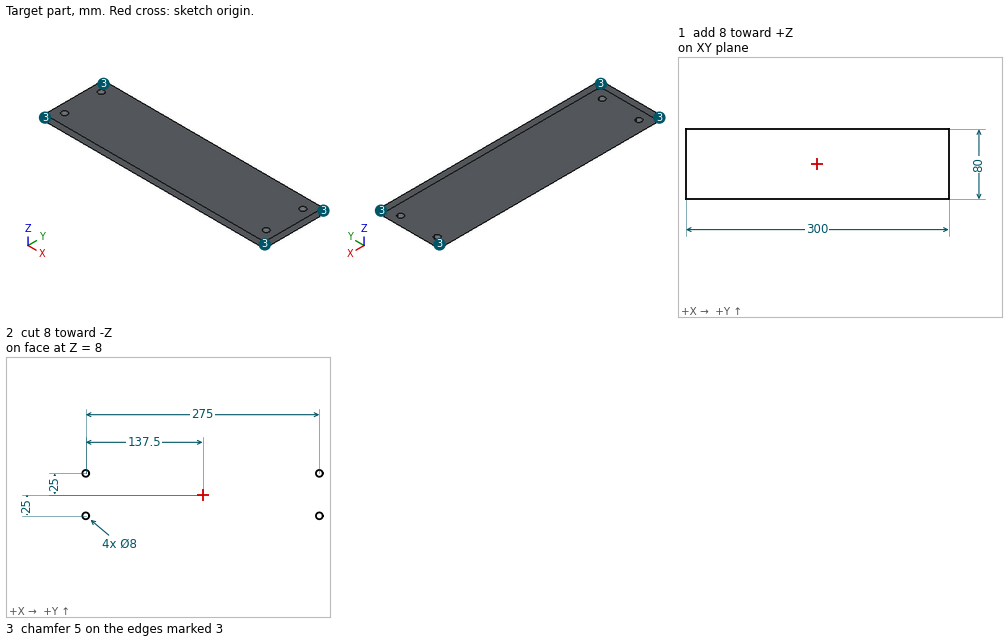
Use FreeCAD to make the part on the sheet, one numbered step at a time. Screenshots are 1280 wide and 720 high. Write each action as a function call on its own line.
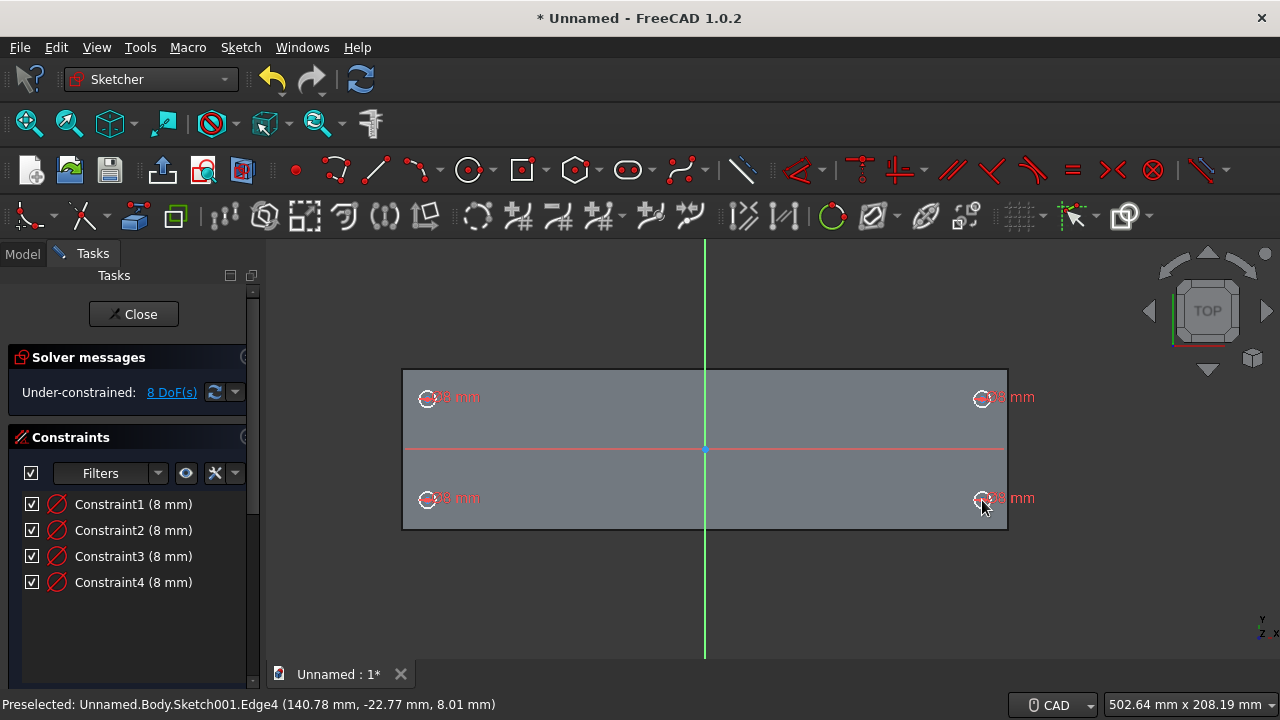
click(428, 399)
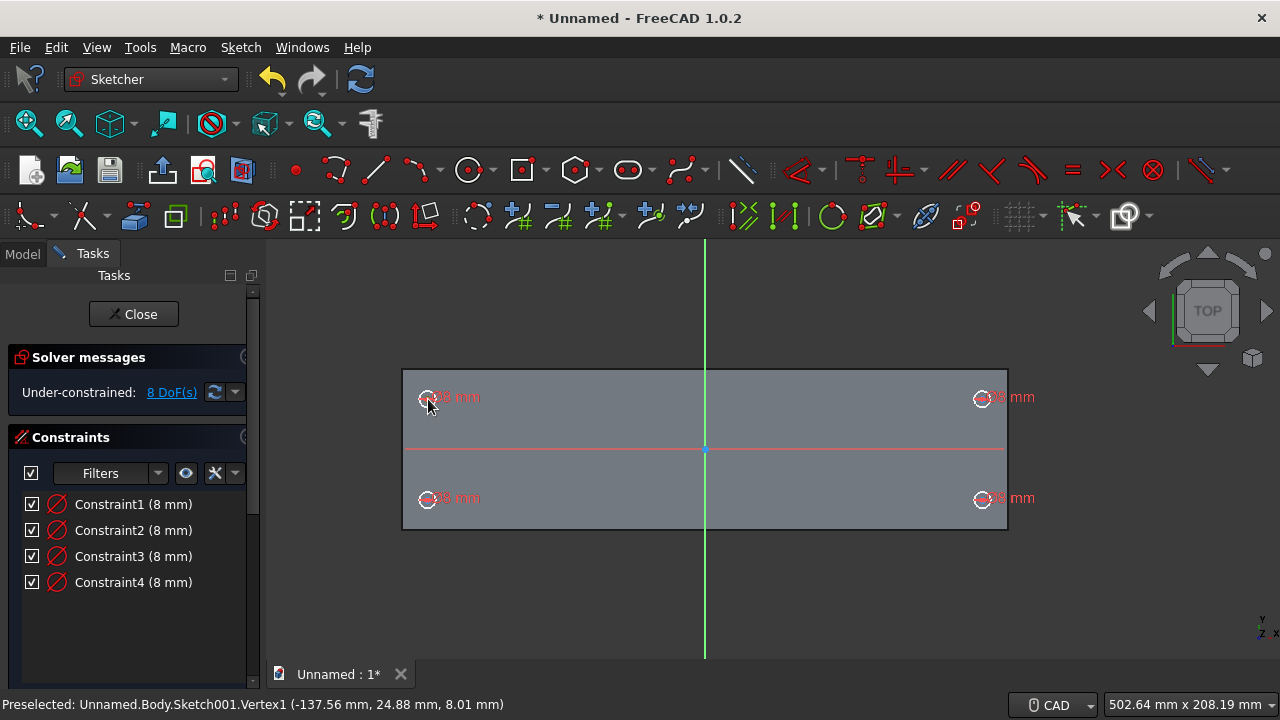
click(428, 500)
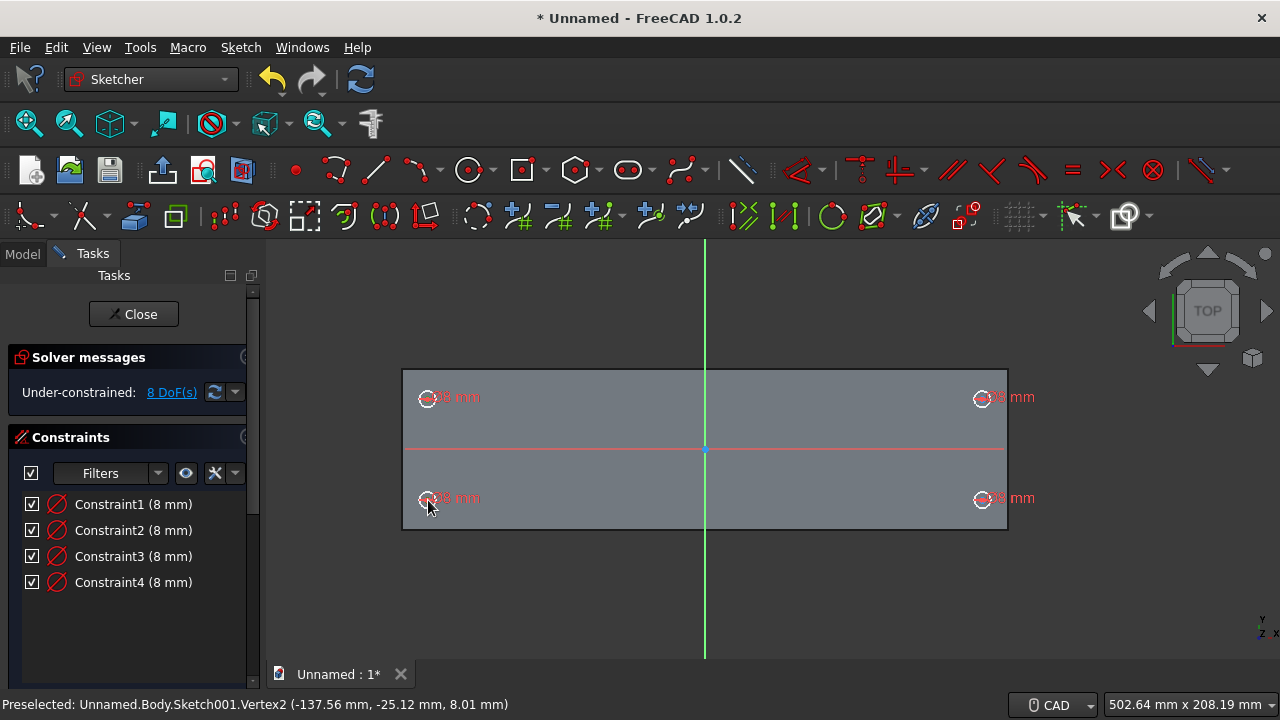
key(v)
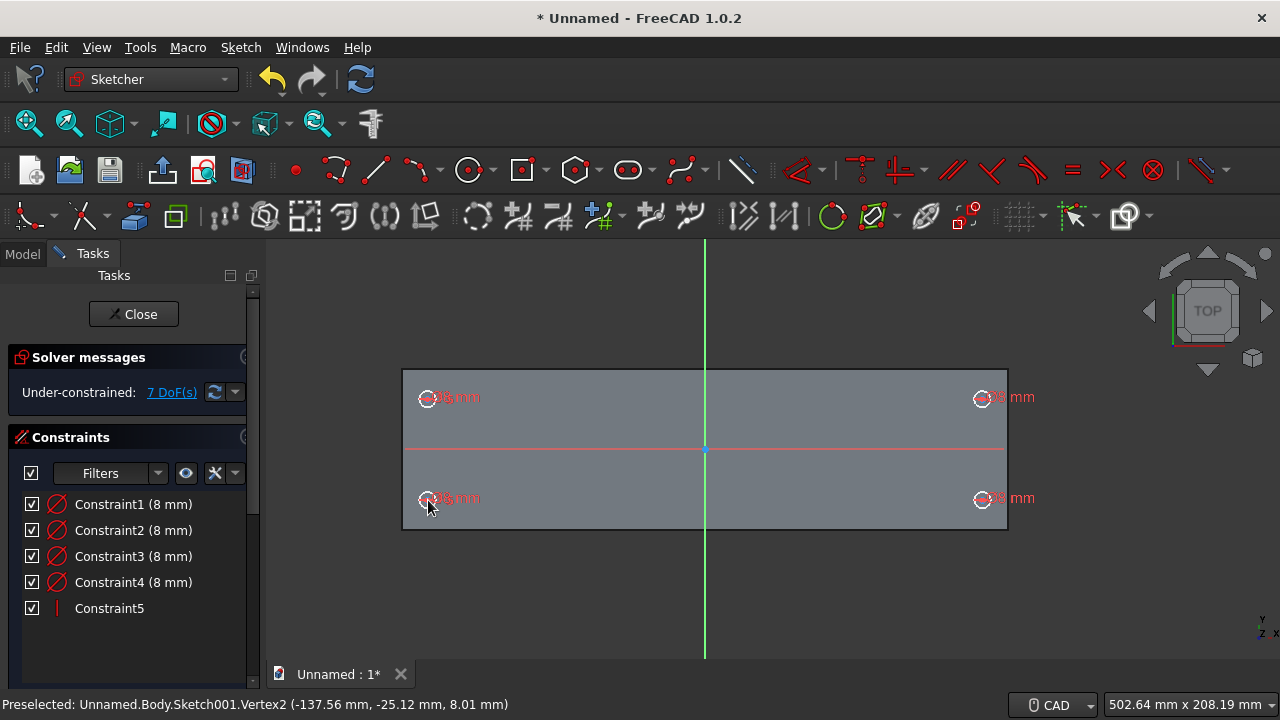
click(428, 399)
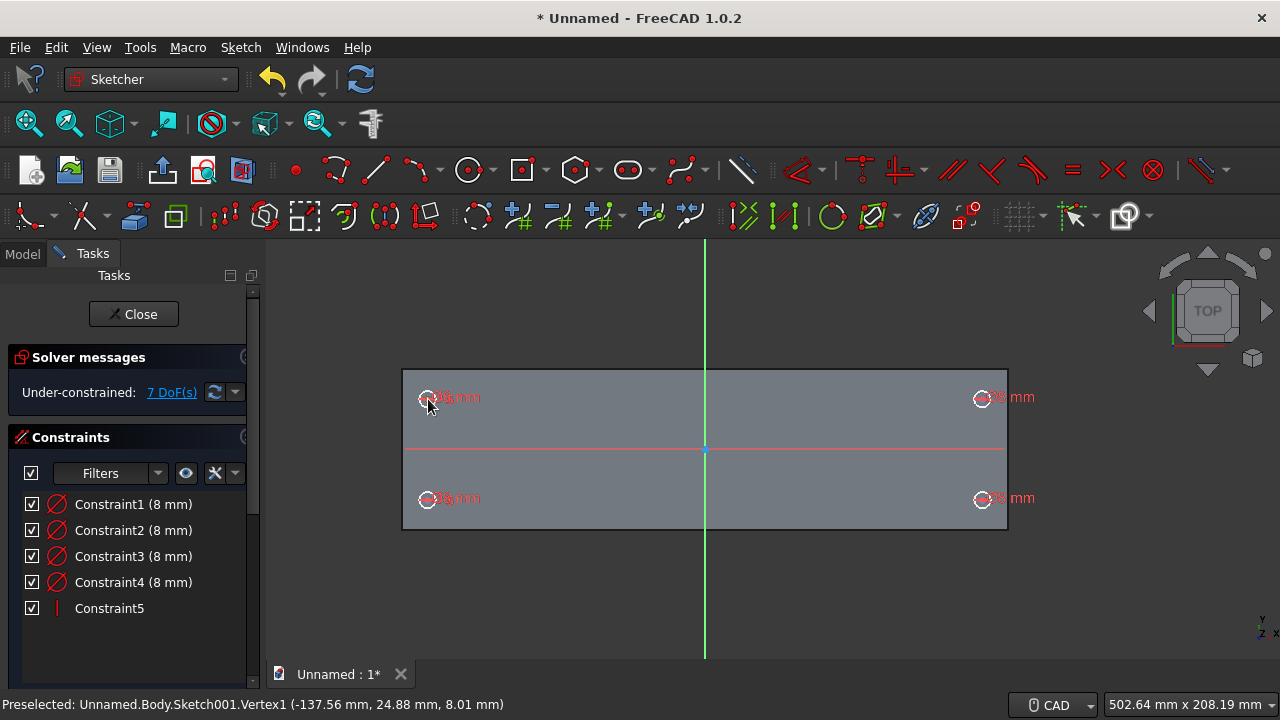
click(982, 399)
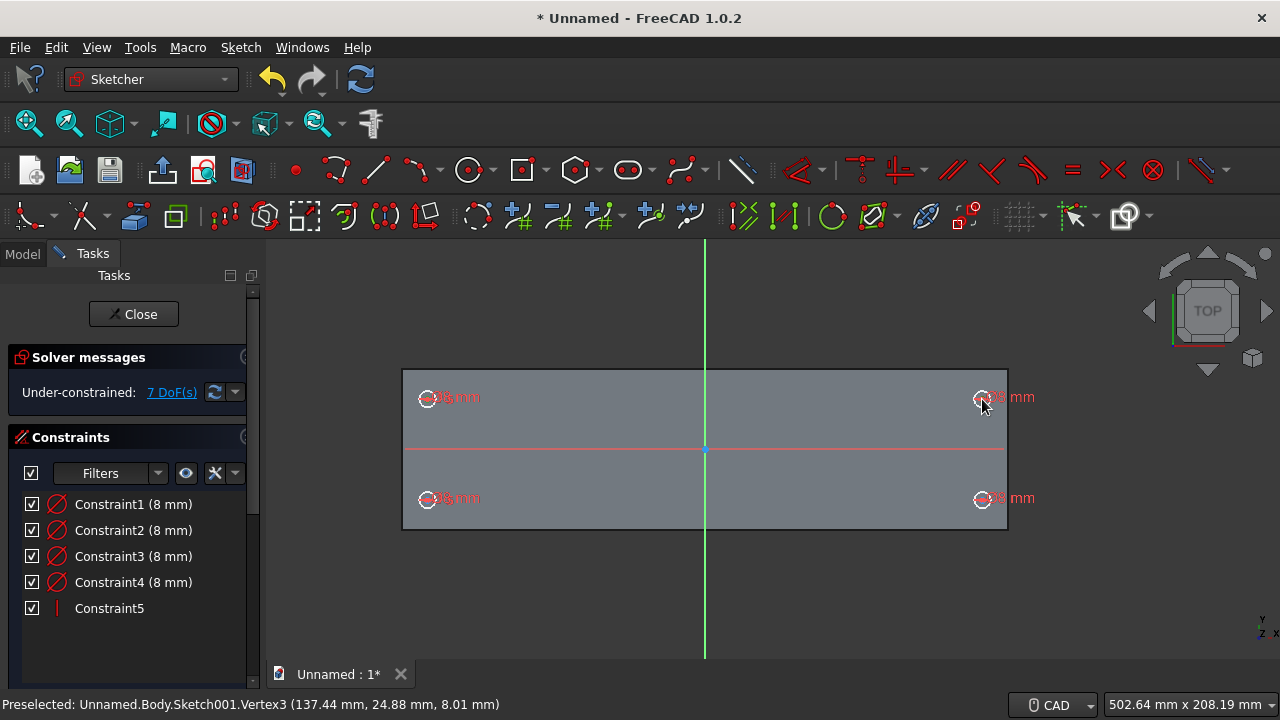
key(h)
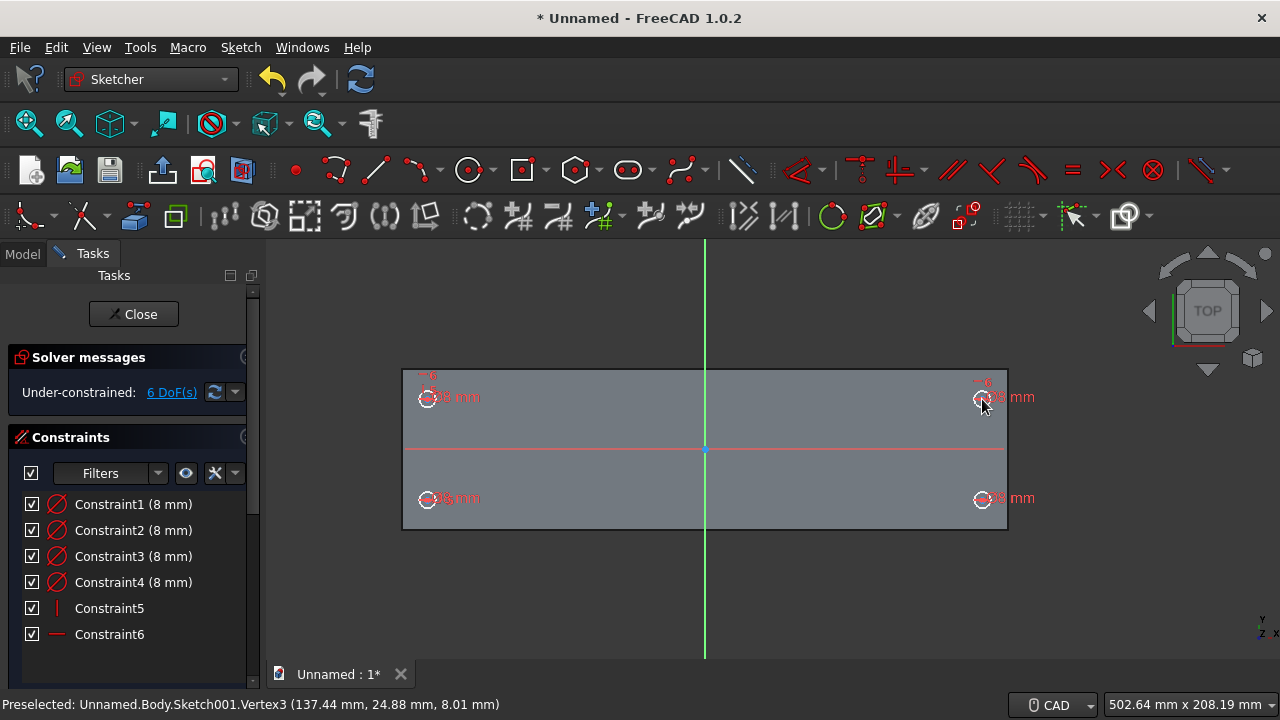
click(982, 399)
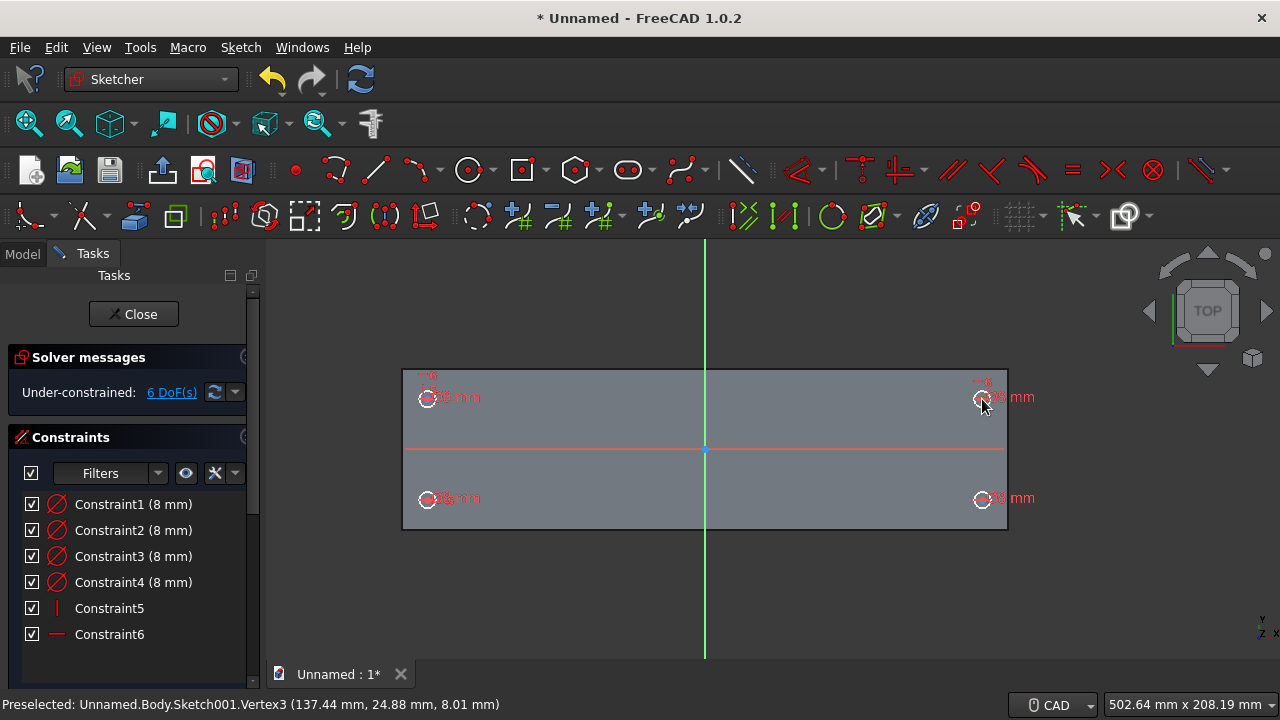
click(982, 500)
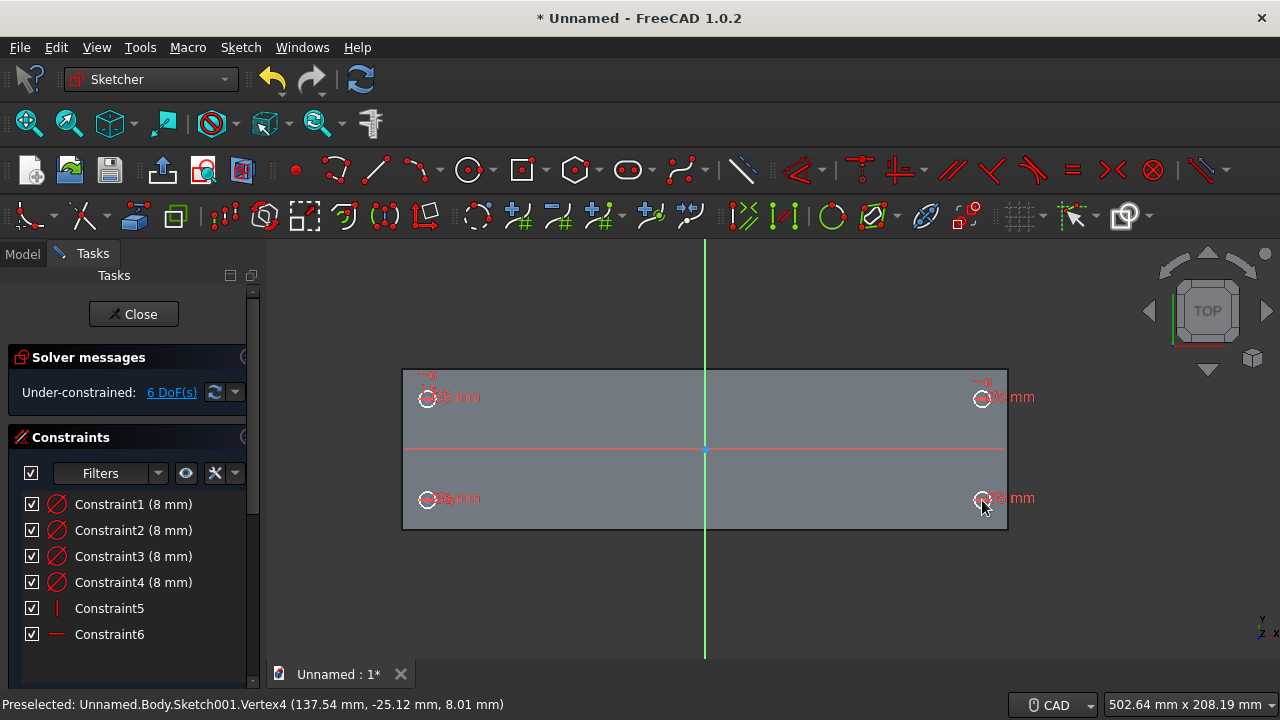
key(v)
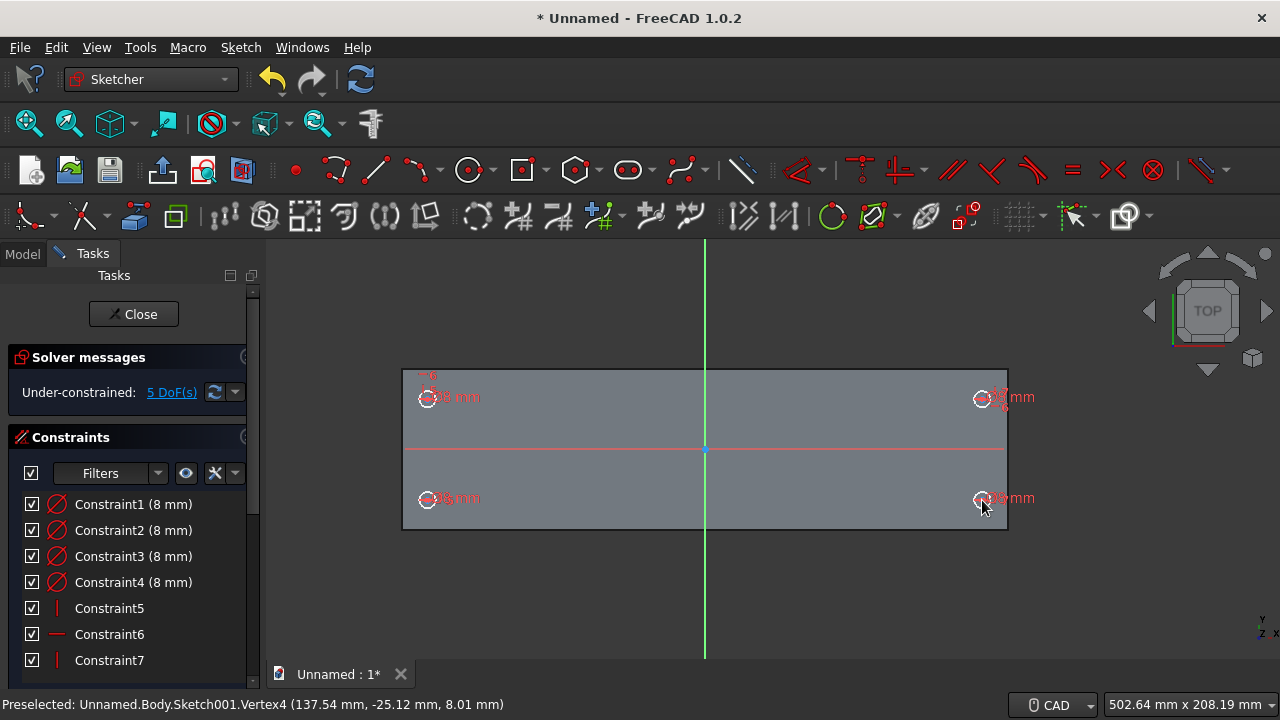
click(428, 500)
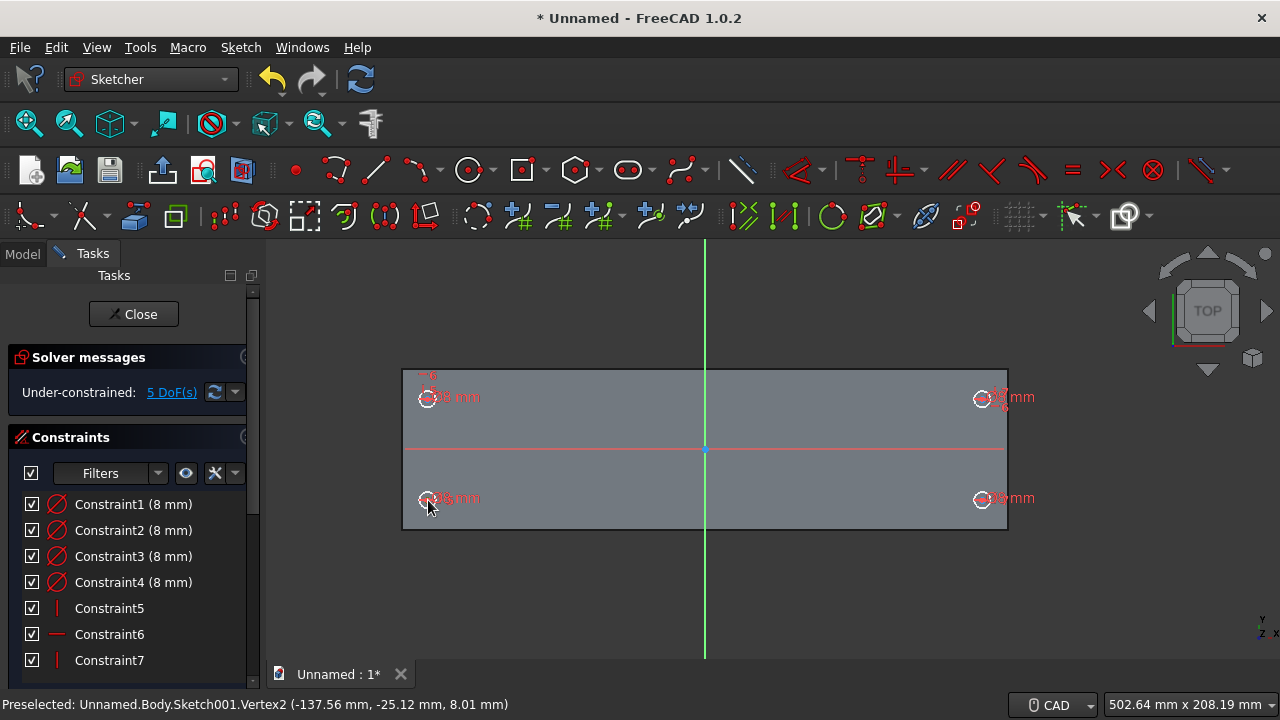
click(982, 500)